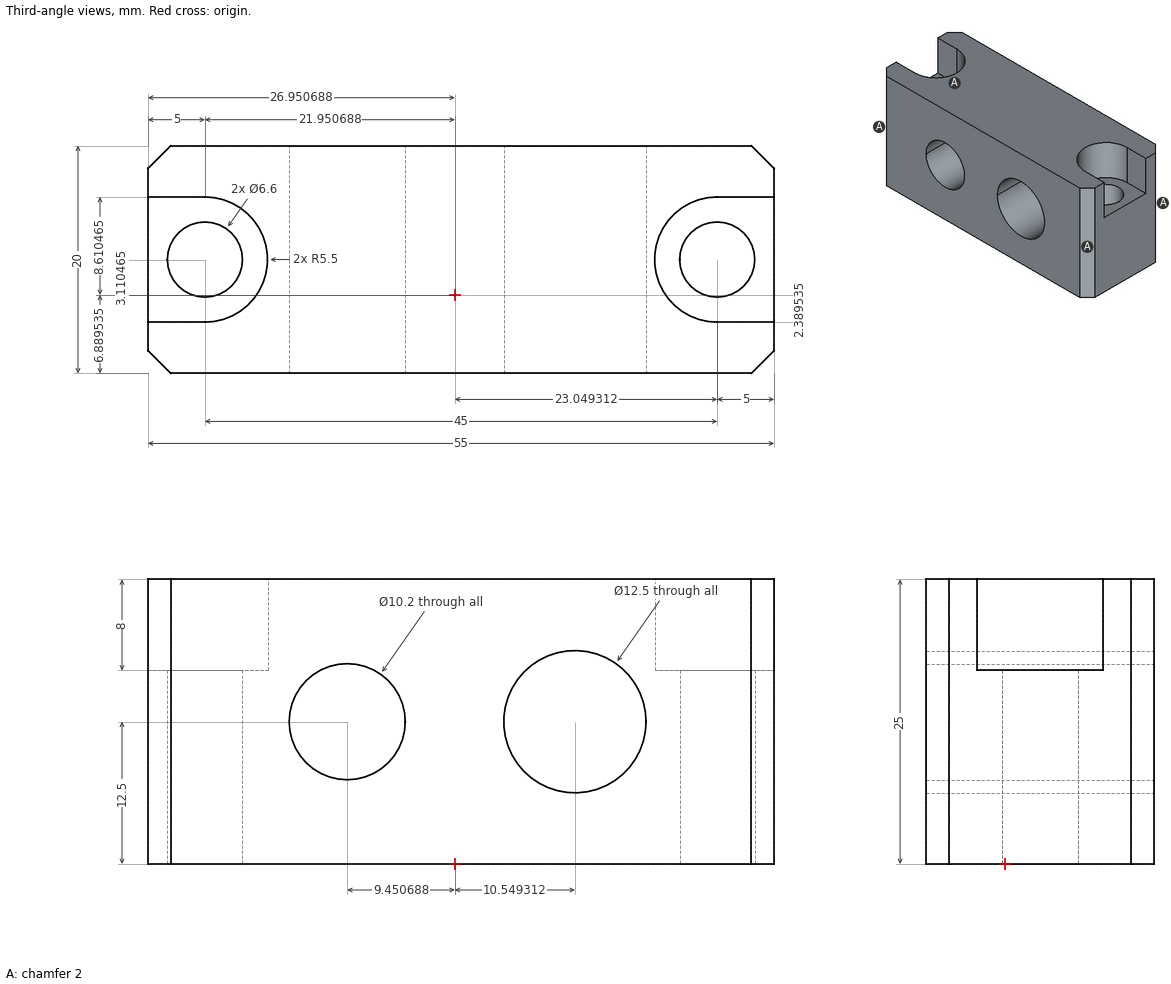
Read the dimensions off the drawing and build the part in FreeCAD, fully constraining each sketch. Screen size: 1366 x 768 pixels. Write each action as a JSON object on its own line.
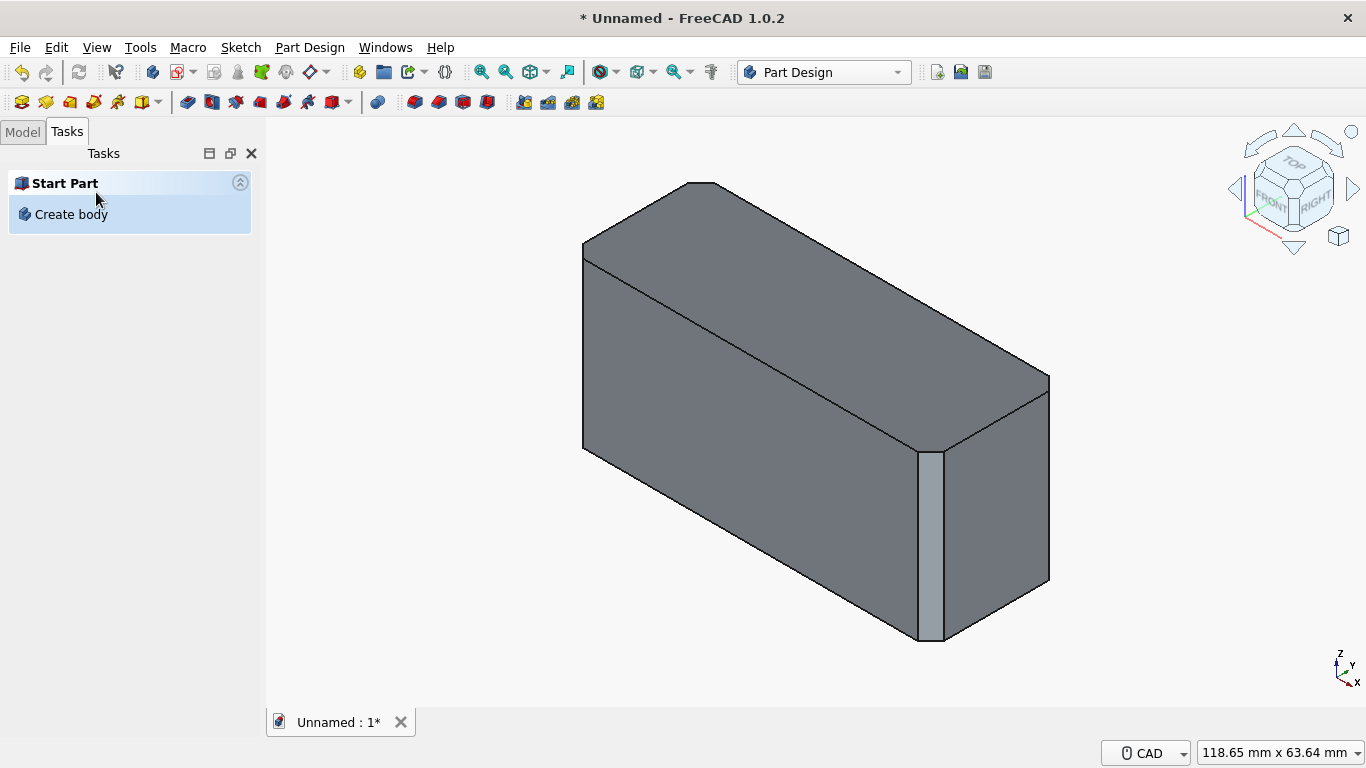
{"action": "left_click", "coordinate": [919, 376]}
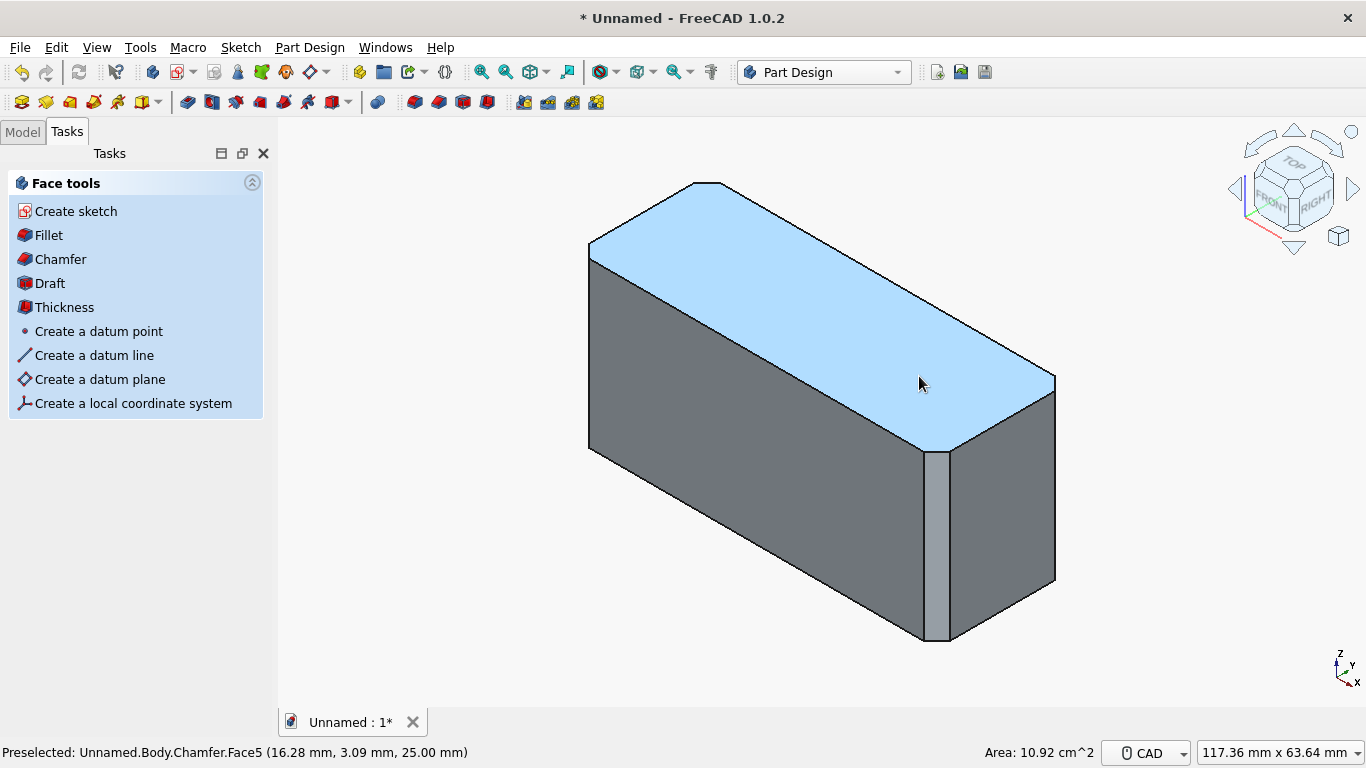
{"action": "left_click", "coordinate": [178, 72]}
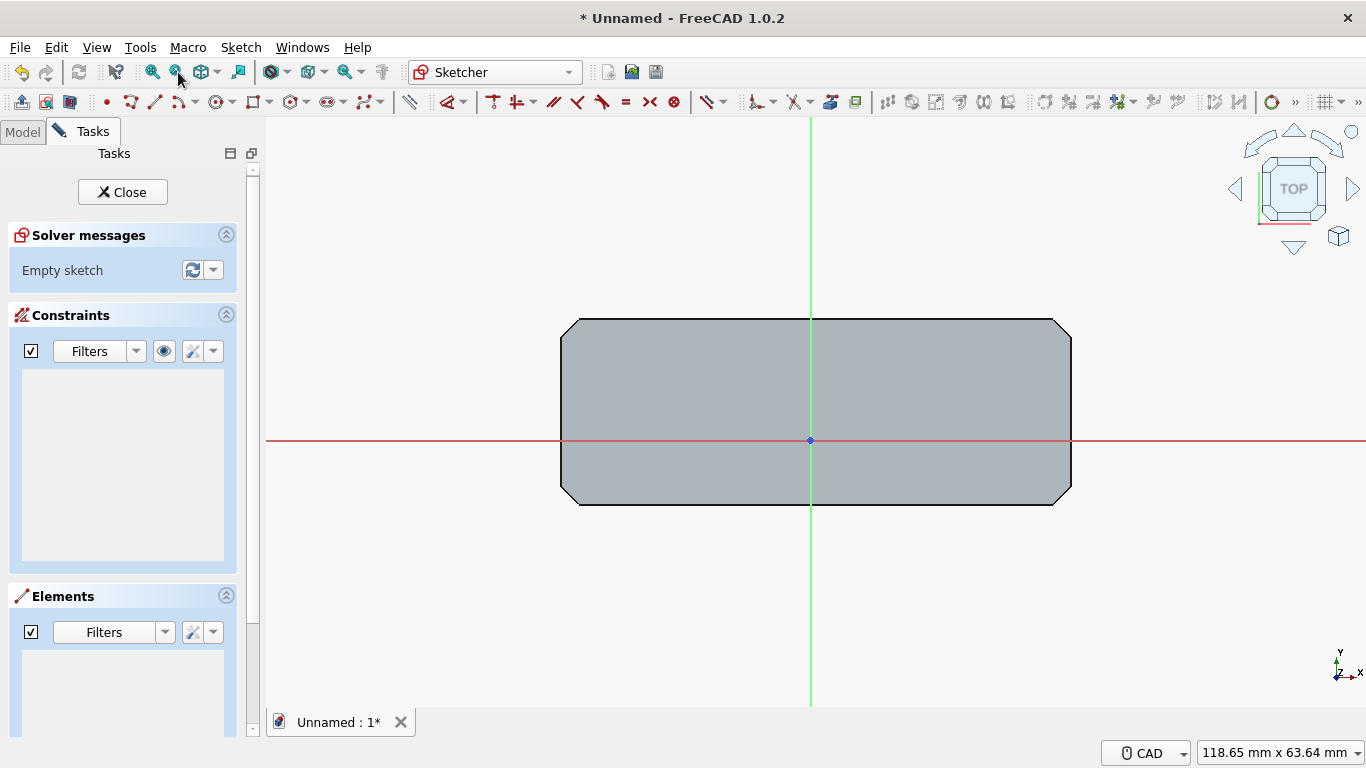
{"action": "left_click", "coordinate": [132, 102]}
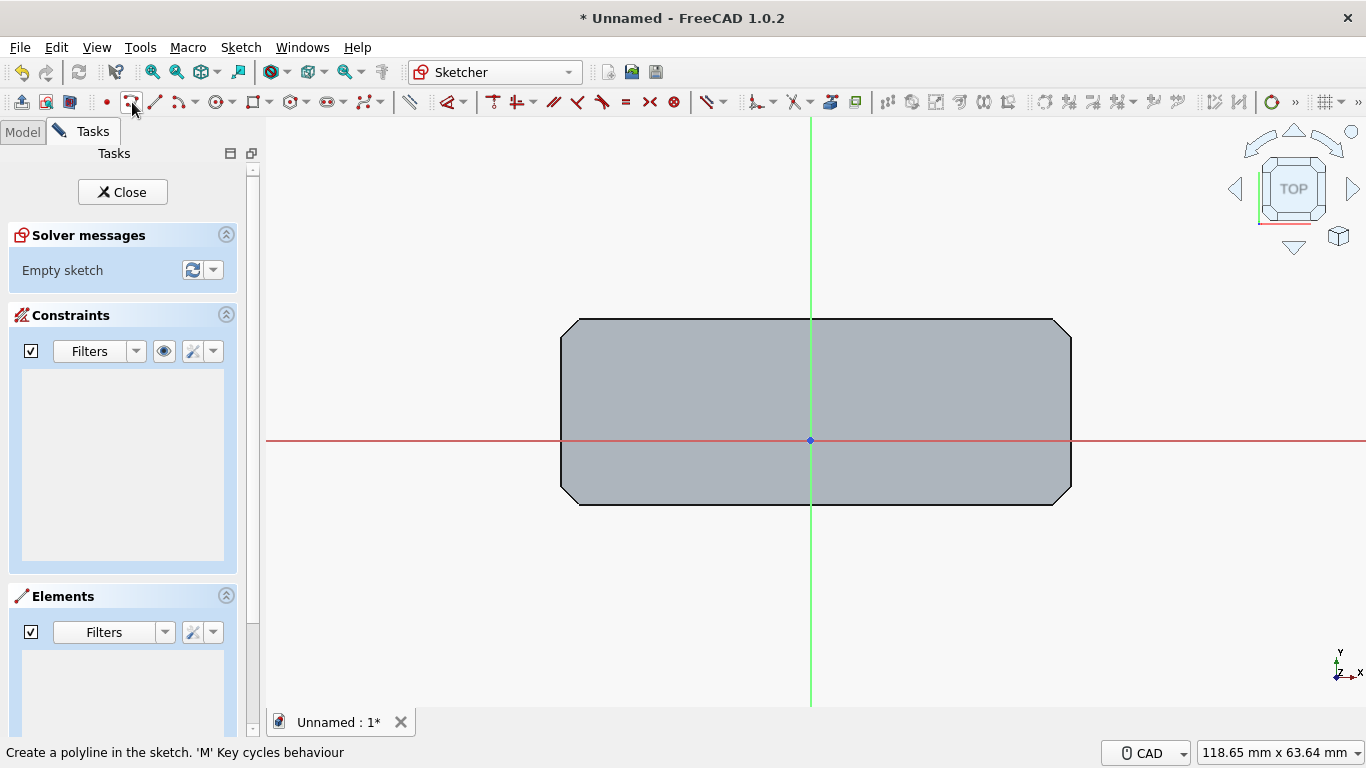
{"action": "left_click", "coordinate": [607, 361]}
{"action": "left_click", "coordinate": [561, 361]}
{"action": "left_click", "coordinate": [561, 463]}
{"action": "left_click", "coordinate": [607, 463]}
{"action": "right_click", "coordinate": [607, 463]}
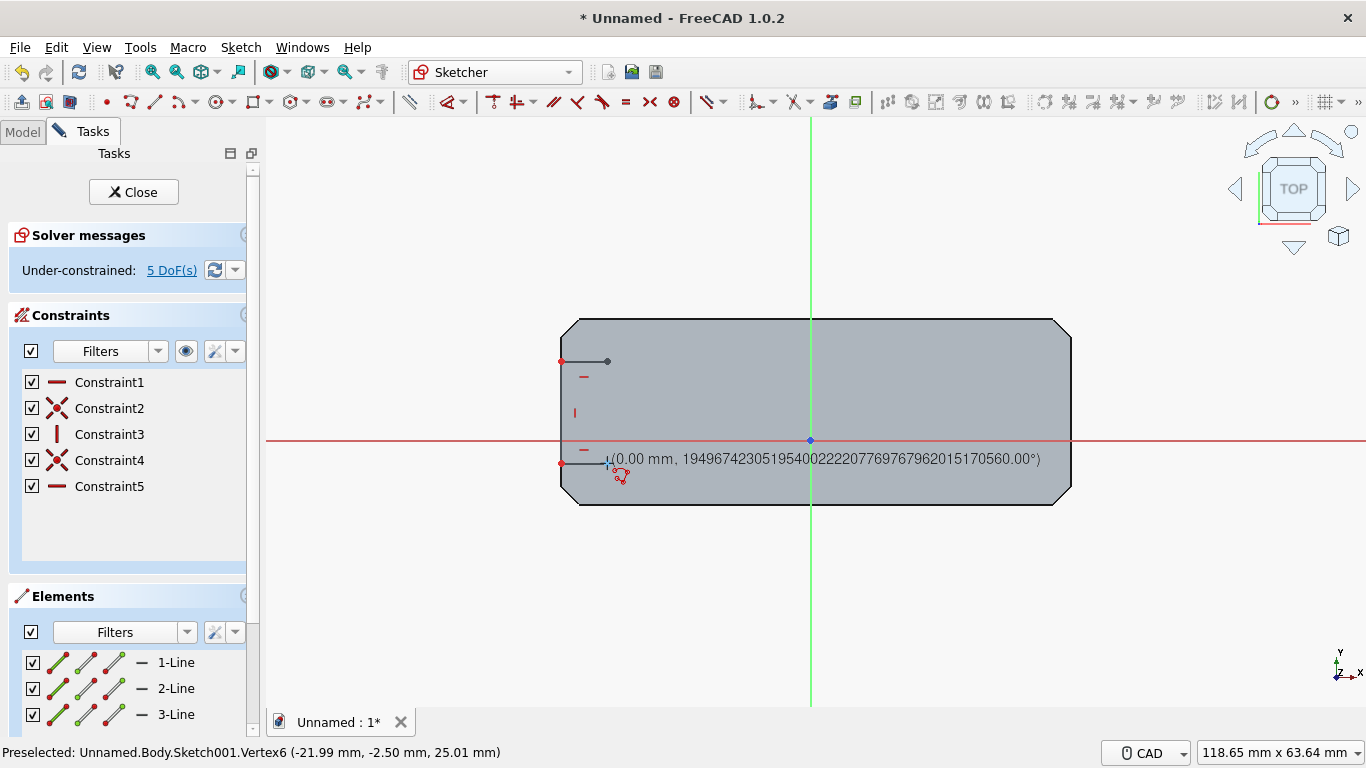
{"action": "left_click", "coordinate": [198, 102]}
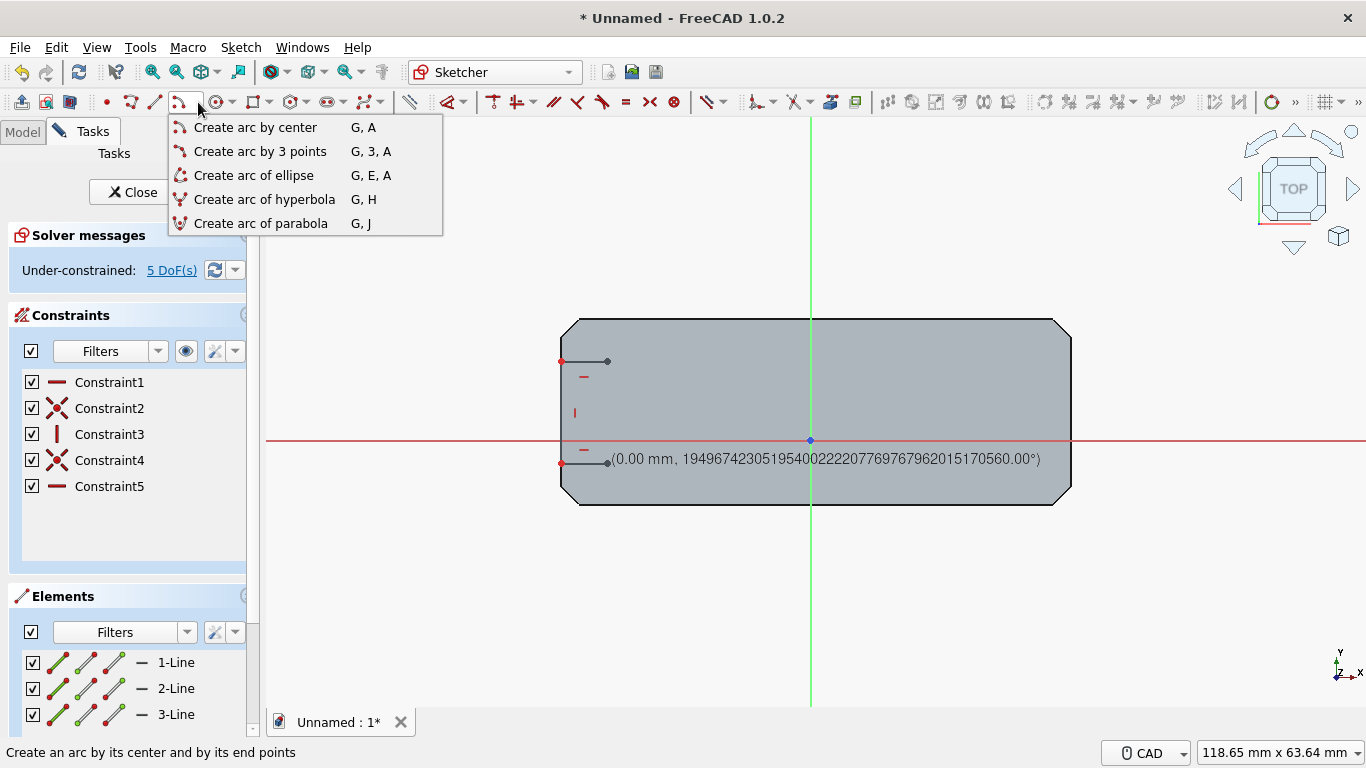
{"action": "left_click", "coordinate": [306, 151]}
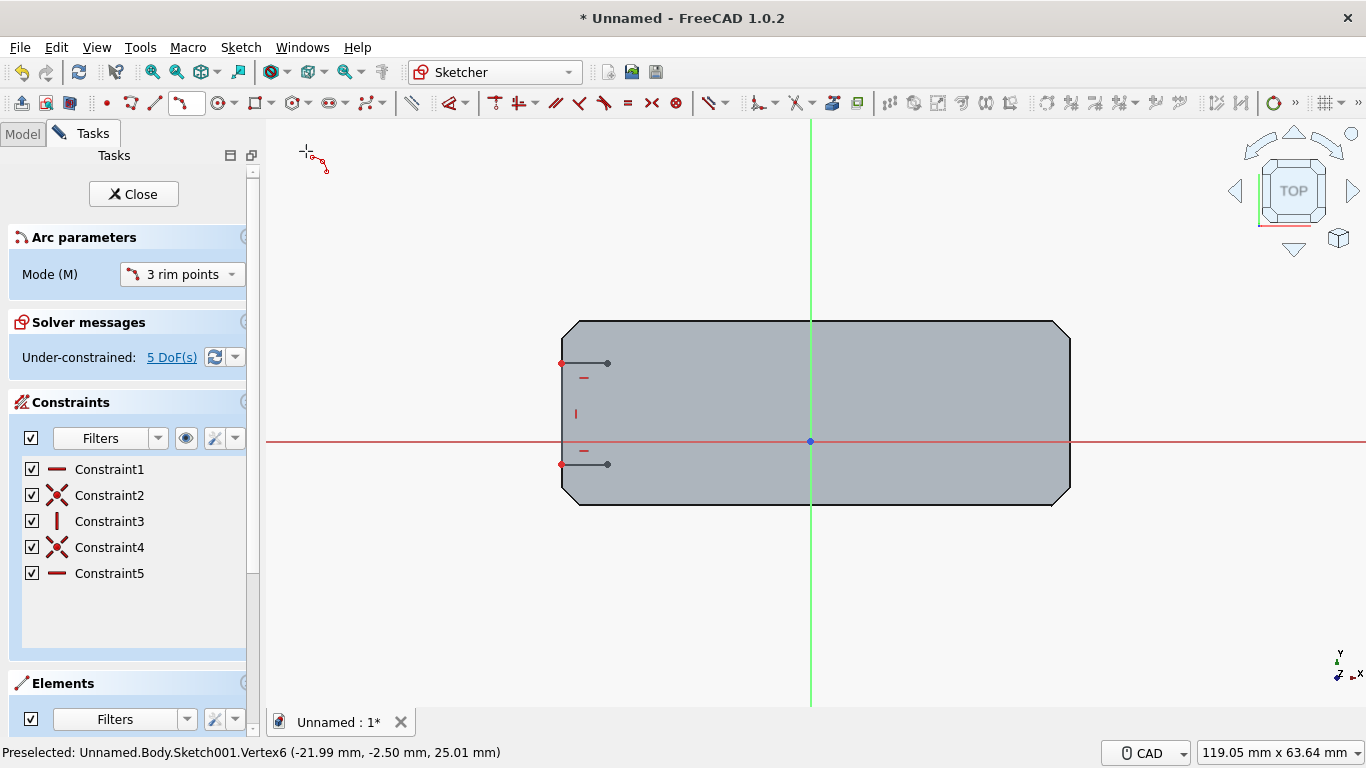
{"action": "left_click", "coordinate": [608, 465]}
{"action": "left_click", "coordinate": [608, 363]}
{"action": "left_click", "coordinate": [659, 413]}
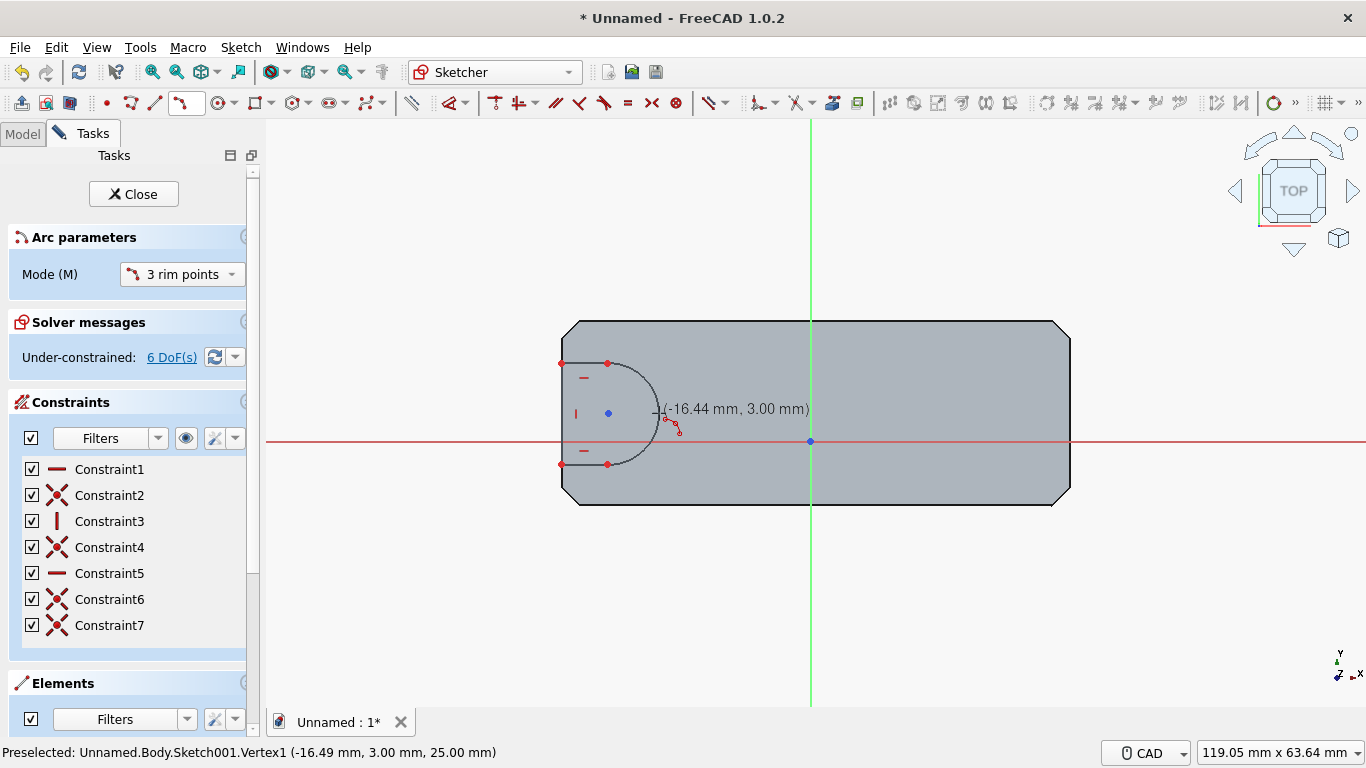
{"action": "left_click", "coordinate": [132, 104]}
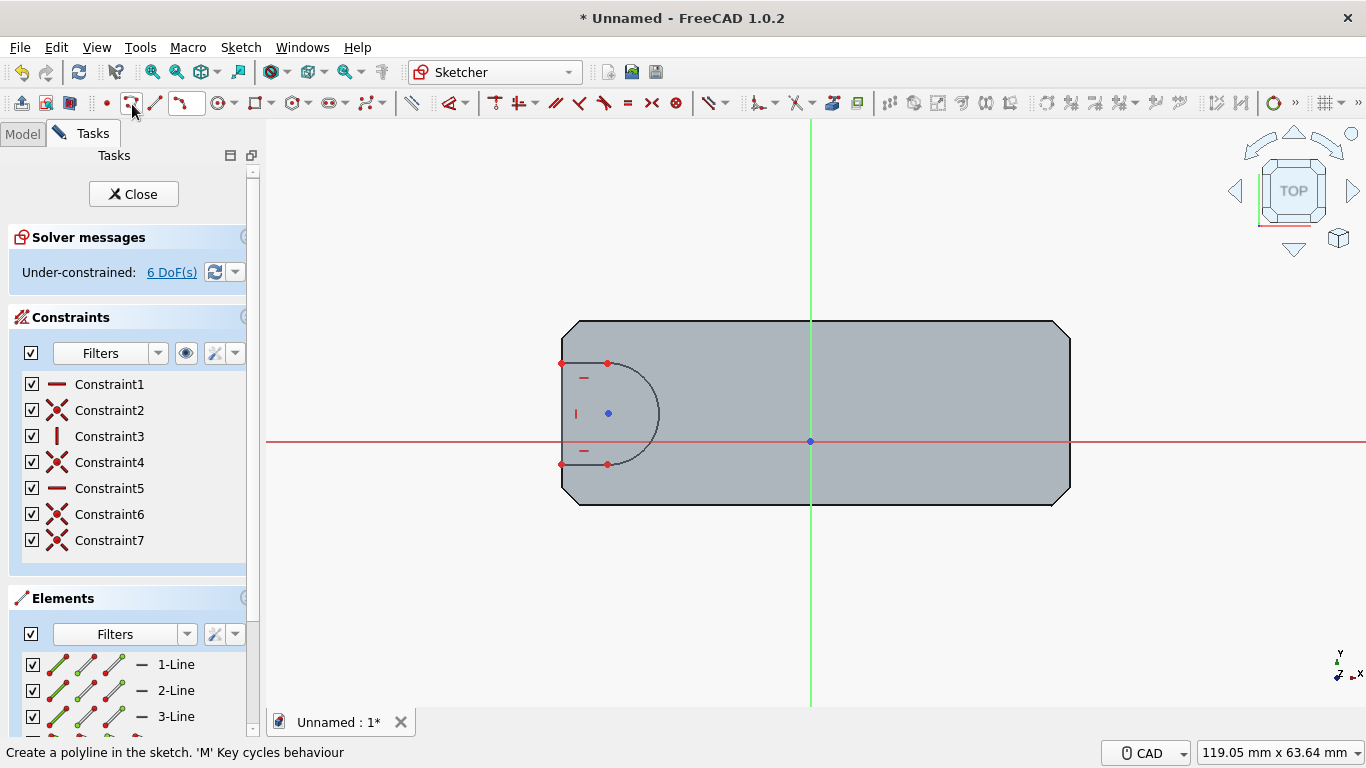
{"action": "left_click", "coordinate": [1024, 464]}
{"action": "left_click", "coordinate": [1070, 464]}
{"action": "left_click", "coordinate": [1070, 362]}
{"action": "left_click", "coordinate": [1024, 362]}
{"action": "right_click", "coordinate": [1024, 362]}